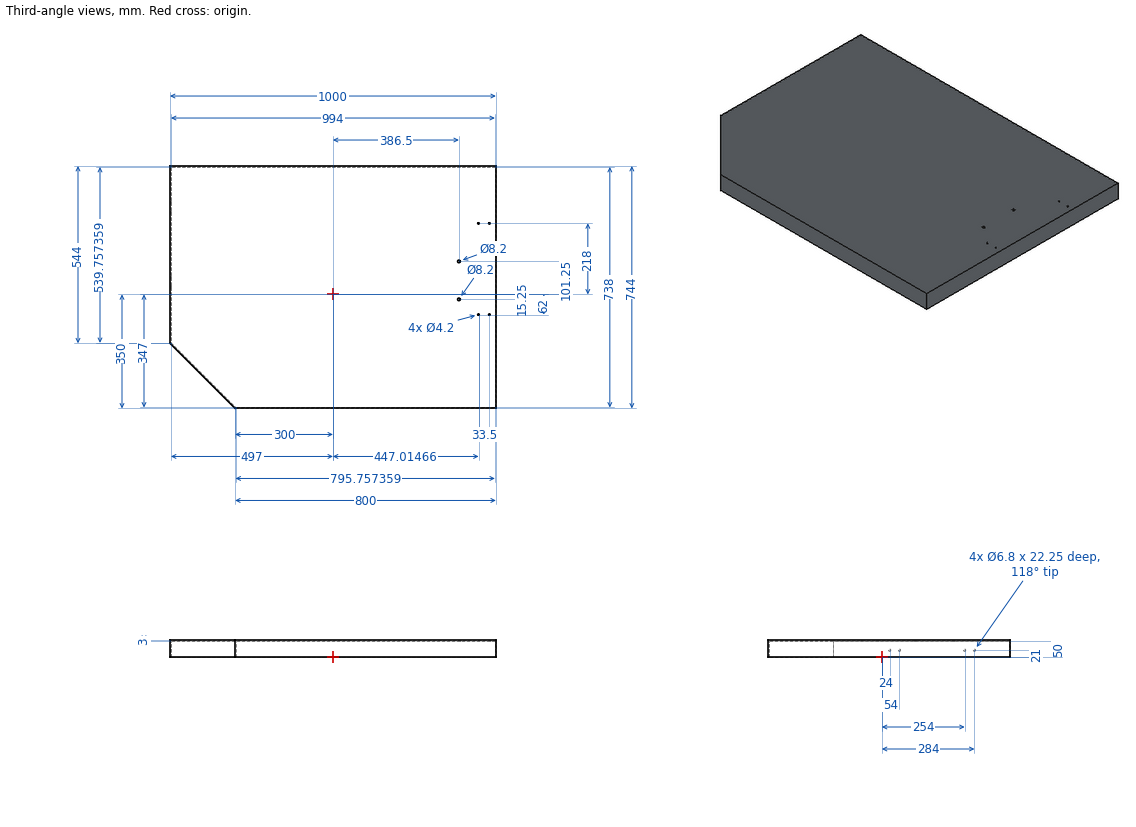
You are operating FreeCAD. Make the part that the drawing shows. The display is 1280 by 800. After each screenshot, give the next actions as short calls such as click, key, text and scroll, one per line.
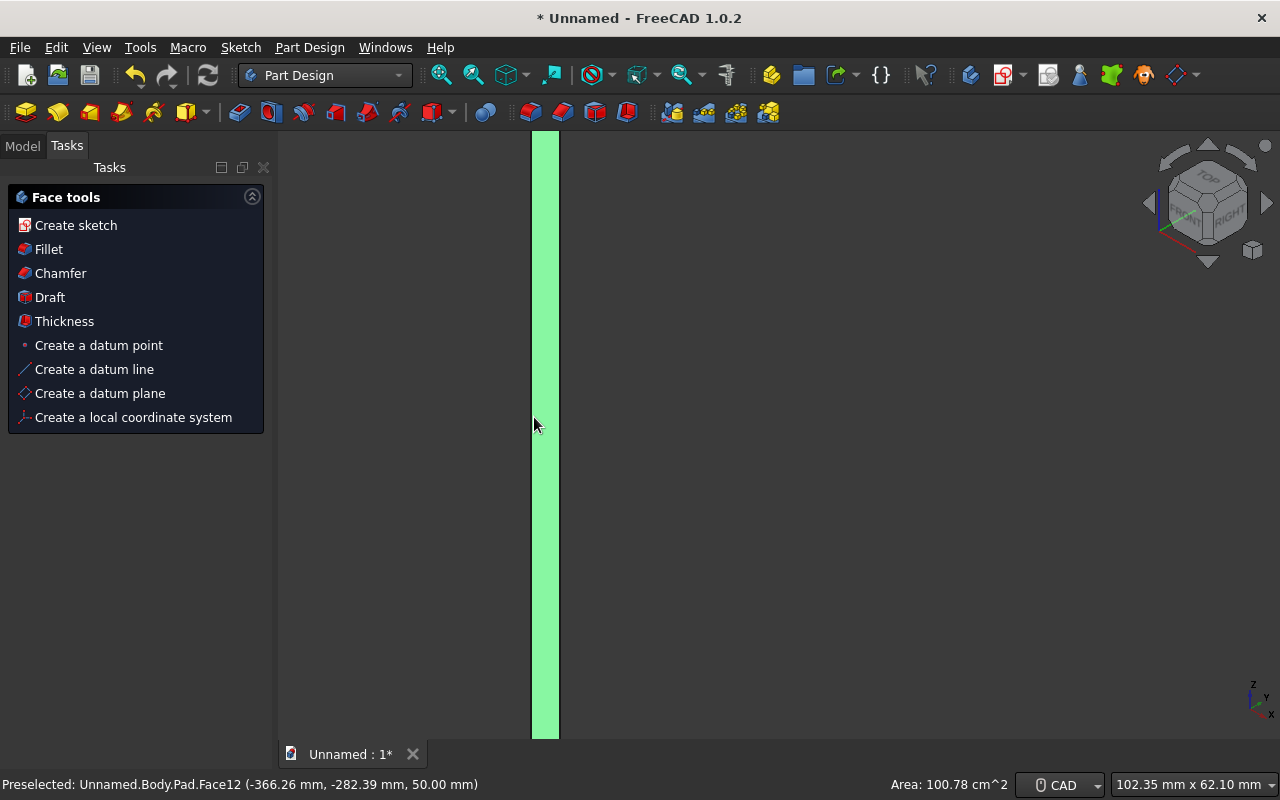
click(1004, 76)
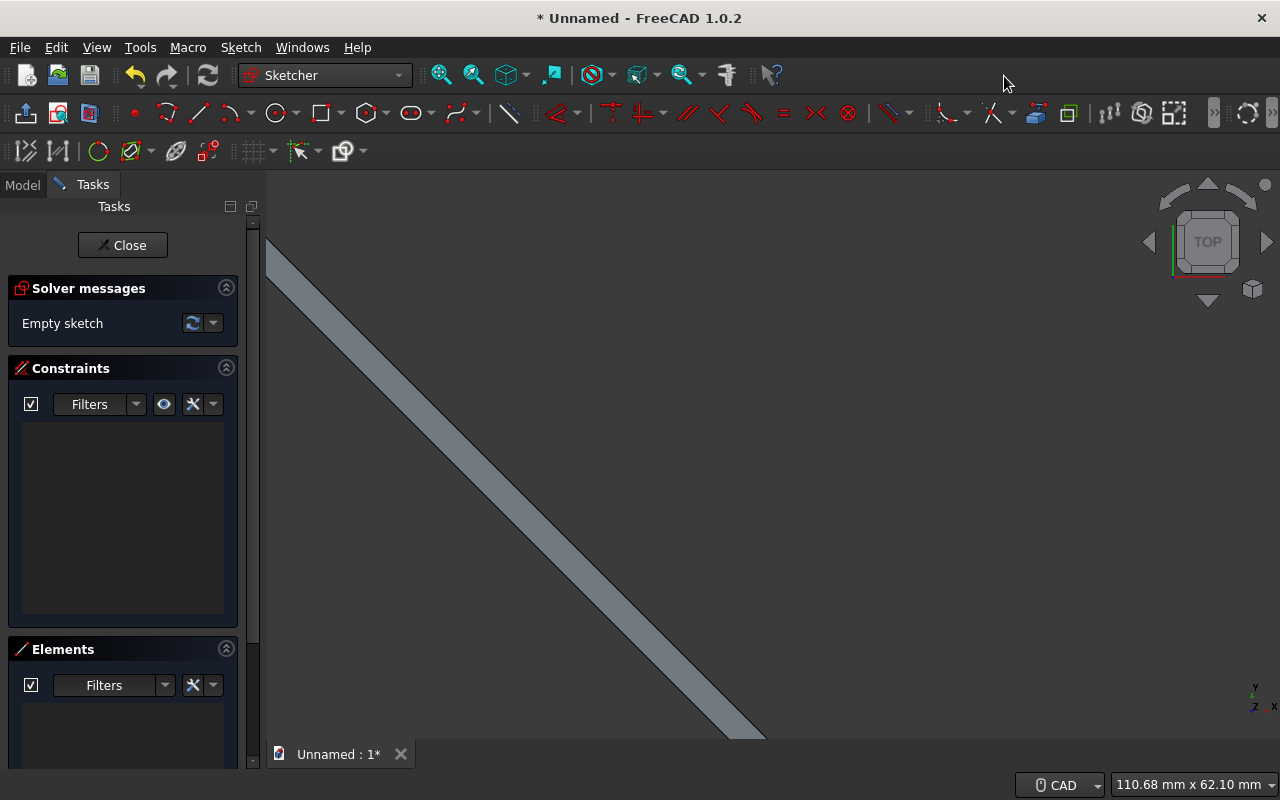
scroll(540, 599, down, 15)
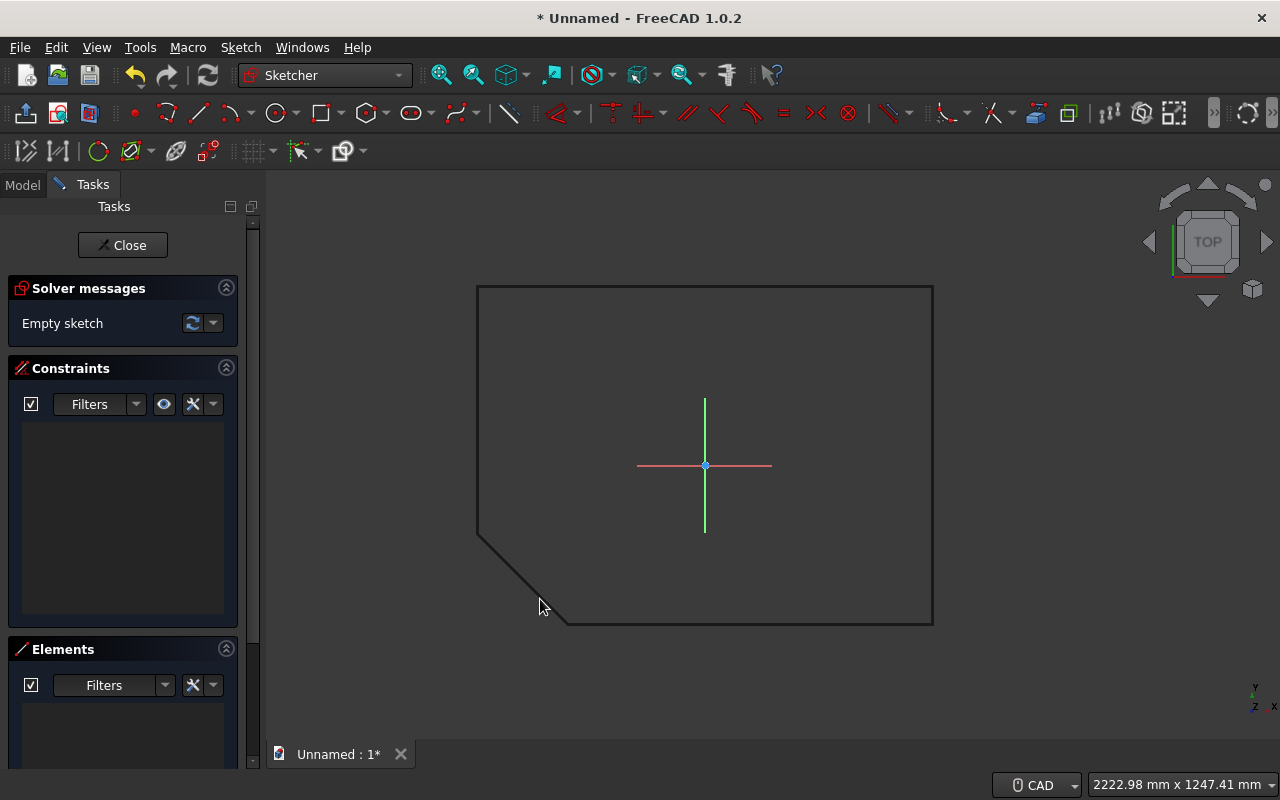
click(168, 114)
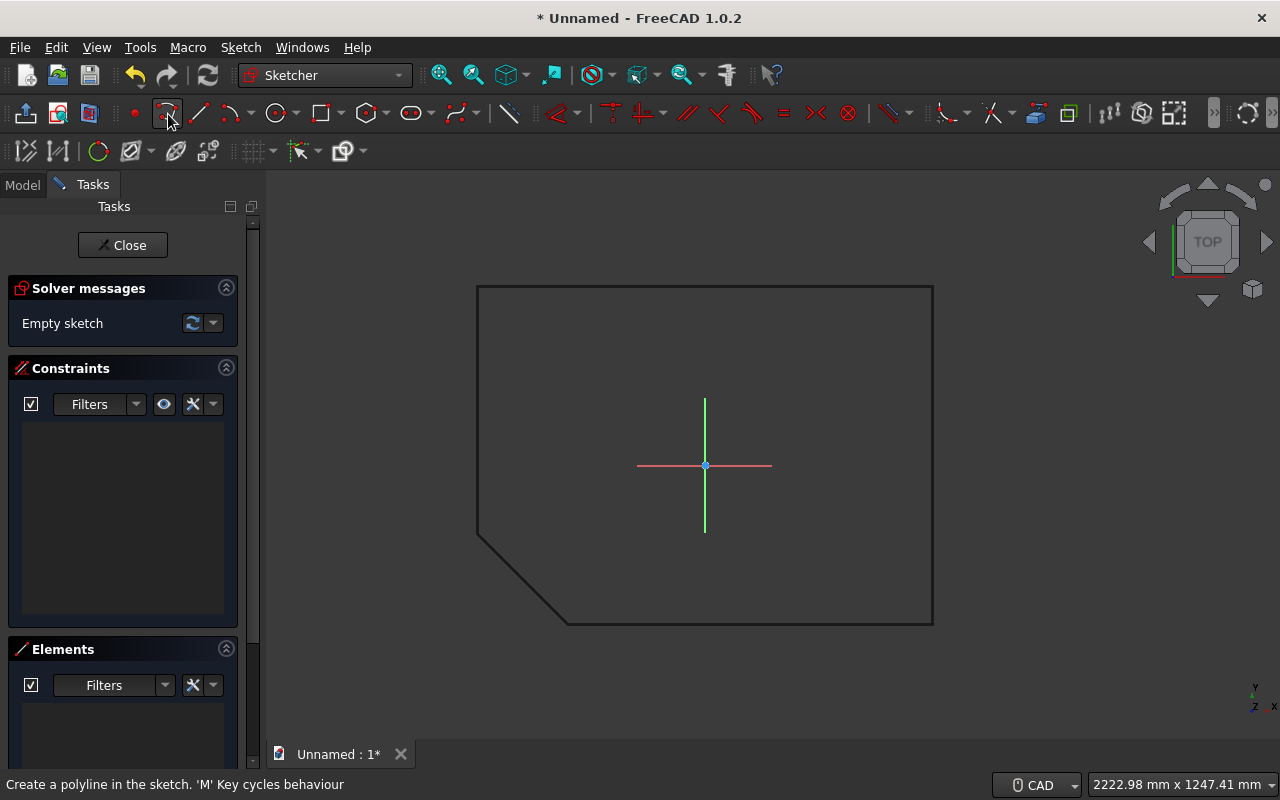
click(568, 625)
click(933, 625)
click(933, 286)
click(477, 286)
click(477, 534)
click(568, 626)
key(Escape)
key(Escape)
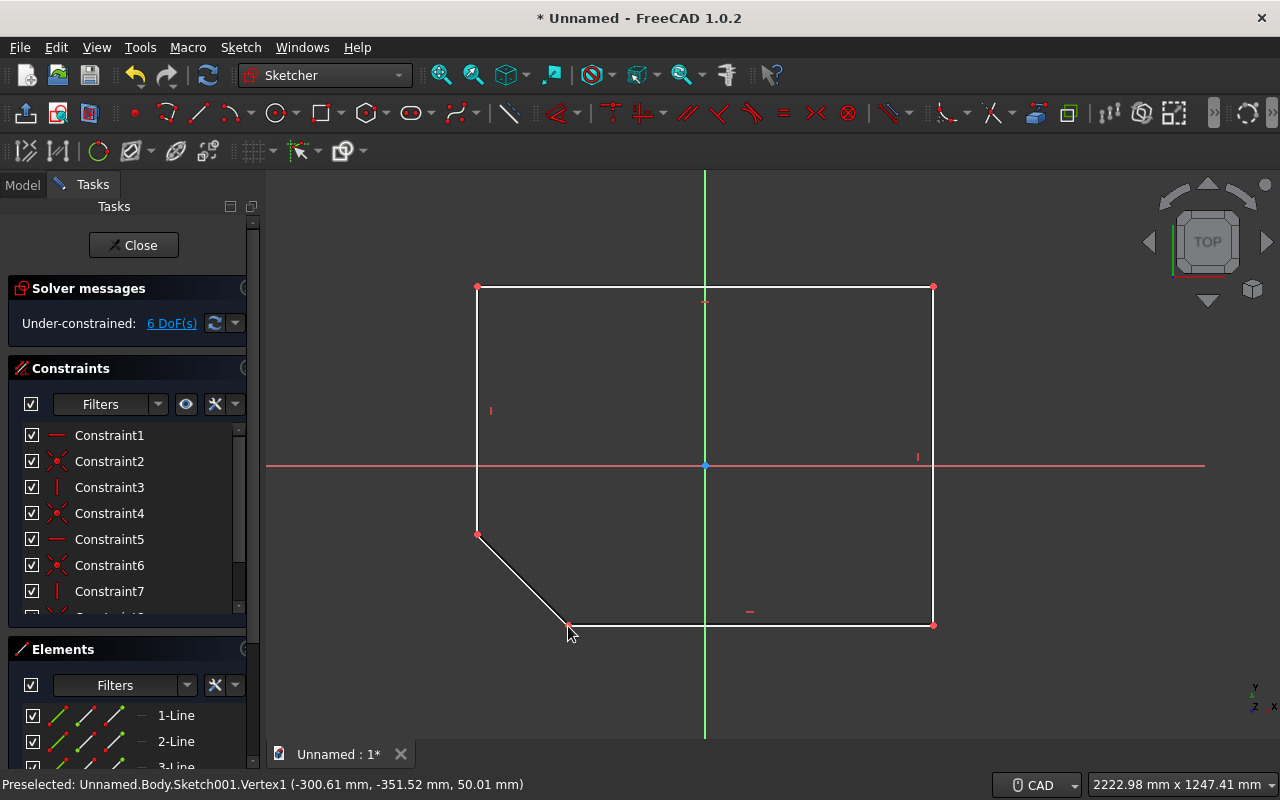
click(556, 114)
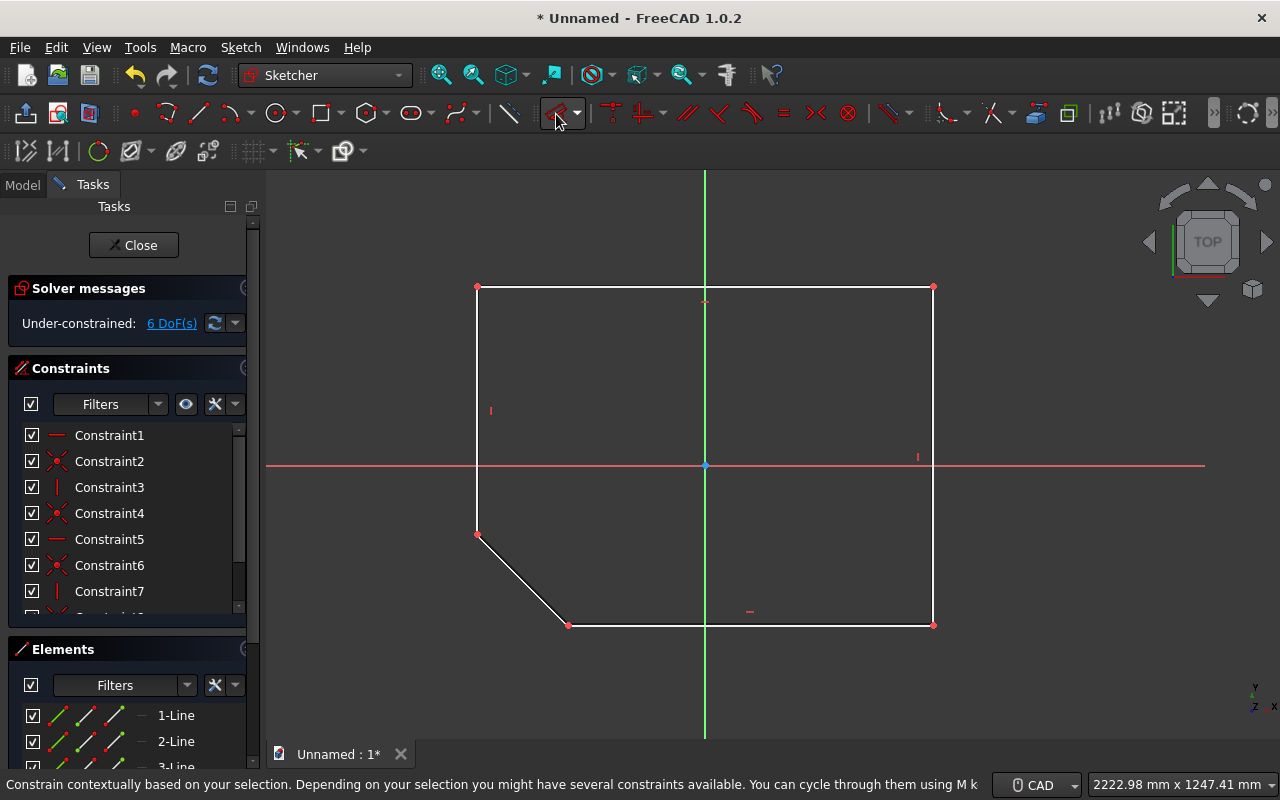
click(677, 626)
click(750, 660)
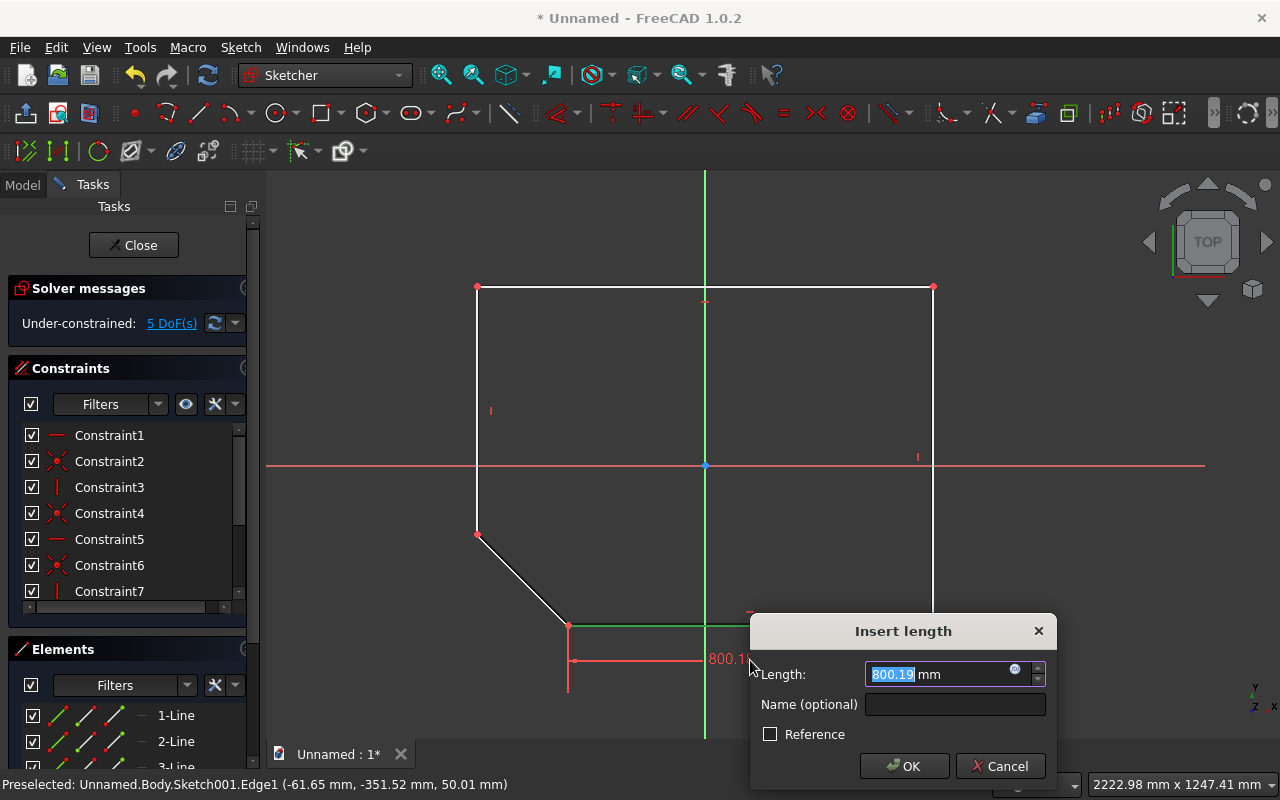
text(800)
key(Return)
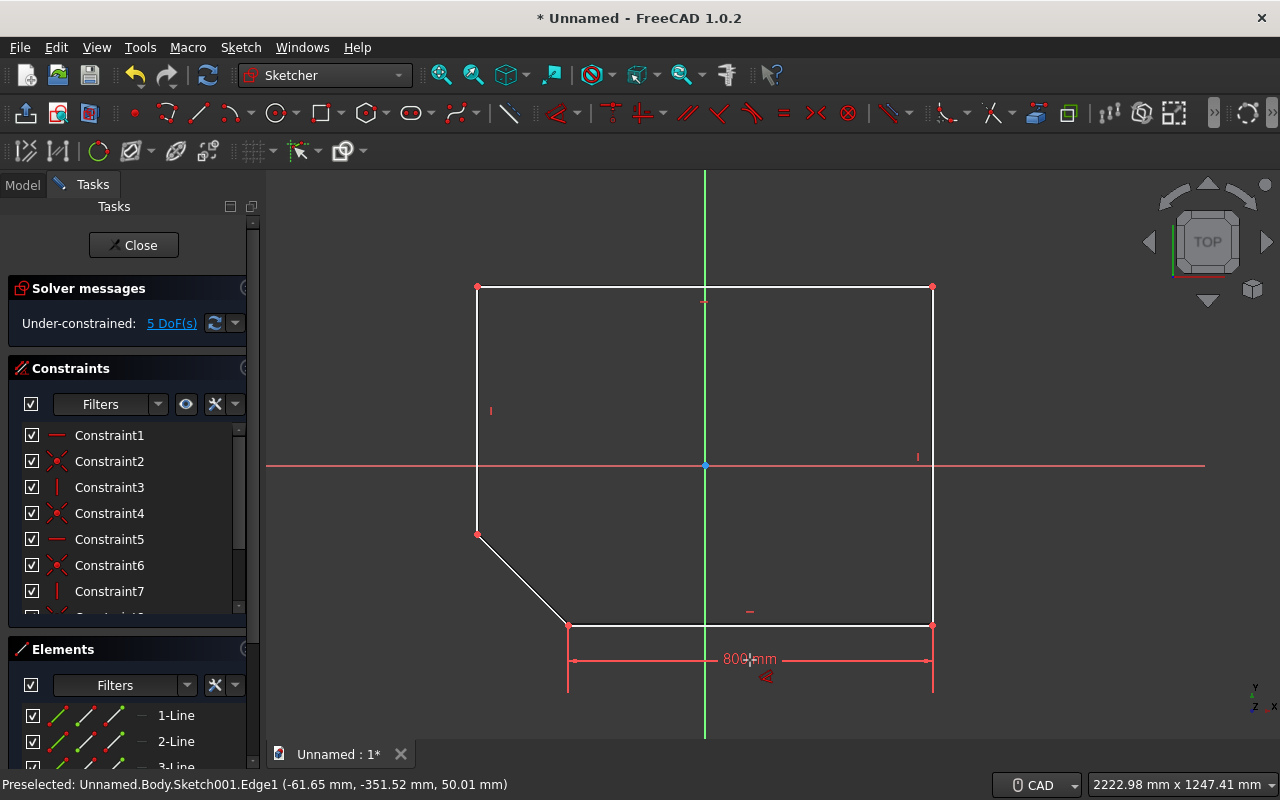
click(933, 524)
click(967, 379)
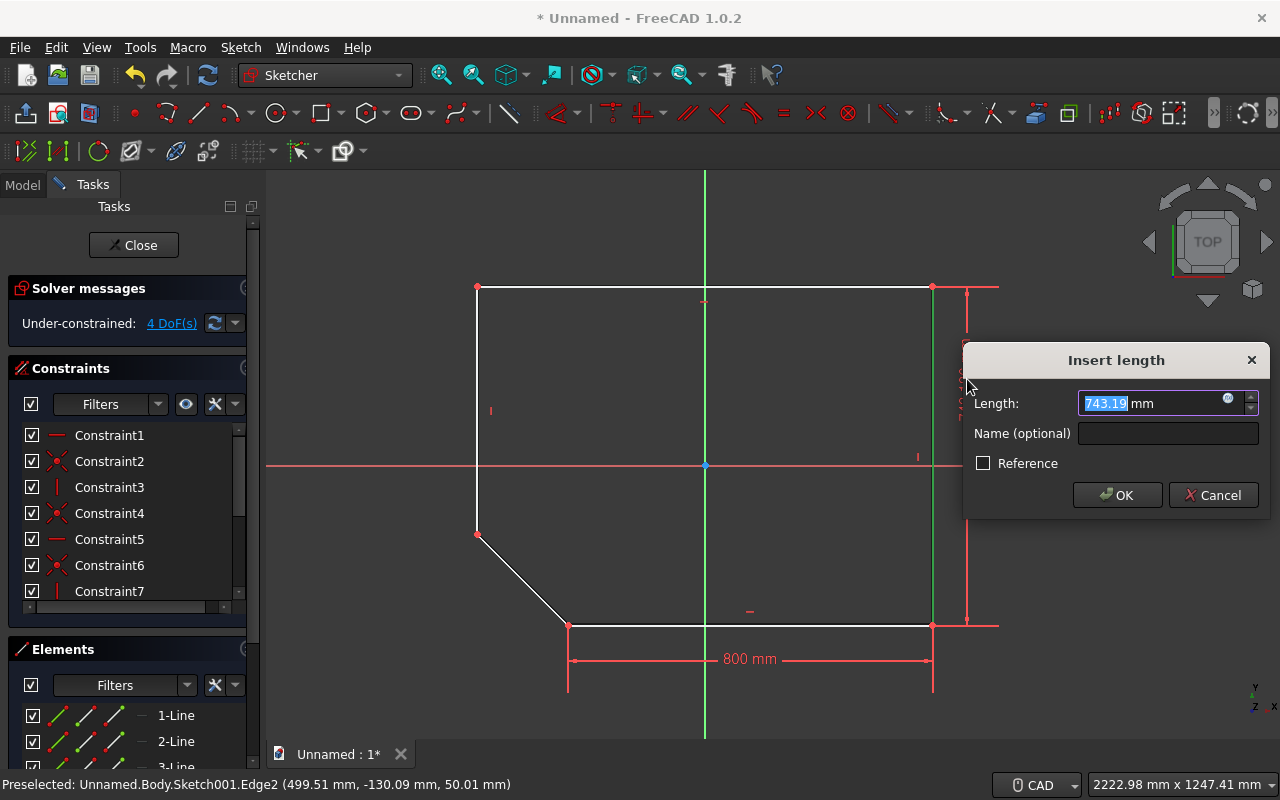
text(744)
key(Return)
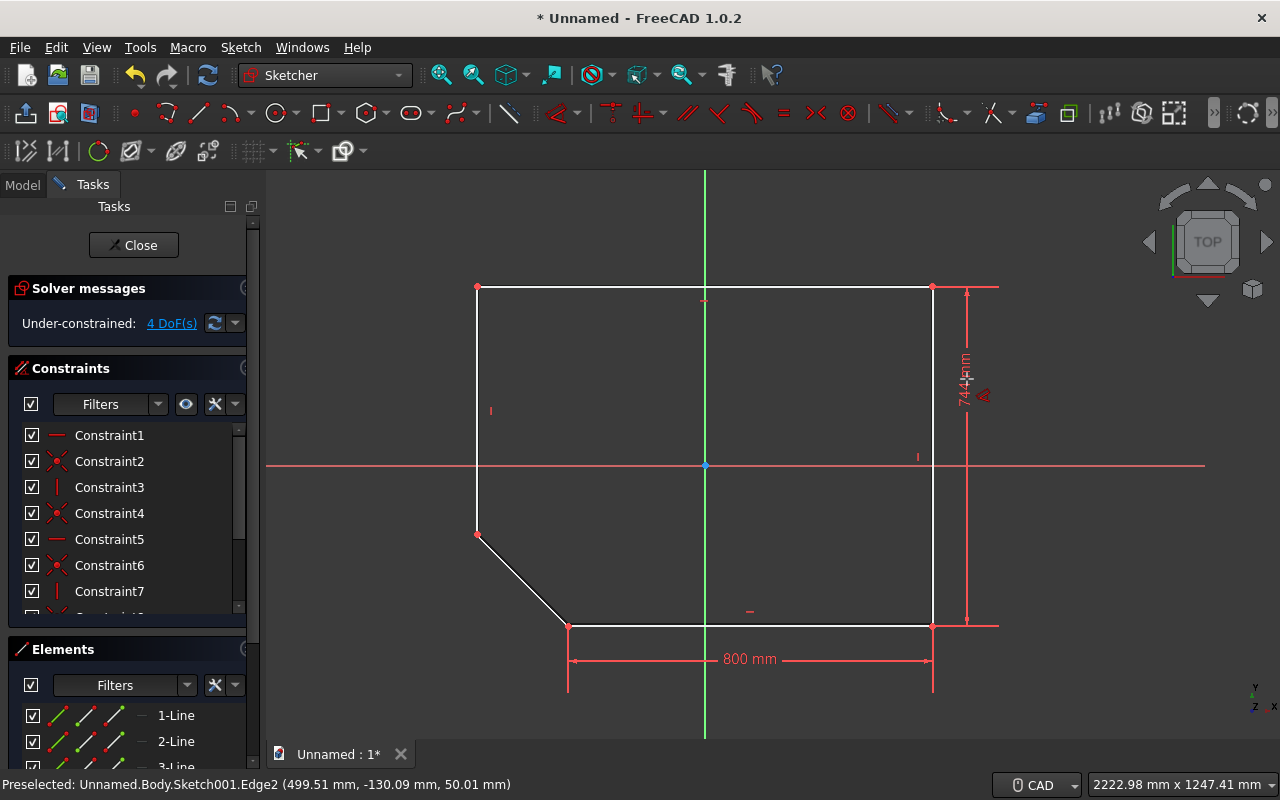
click(477, 361)
click(443, 411)